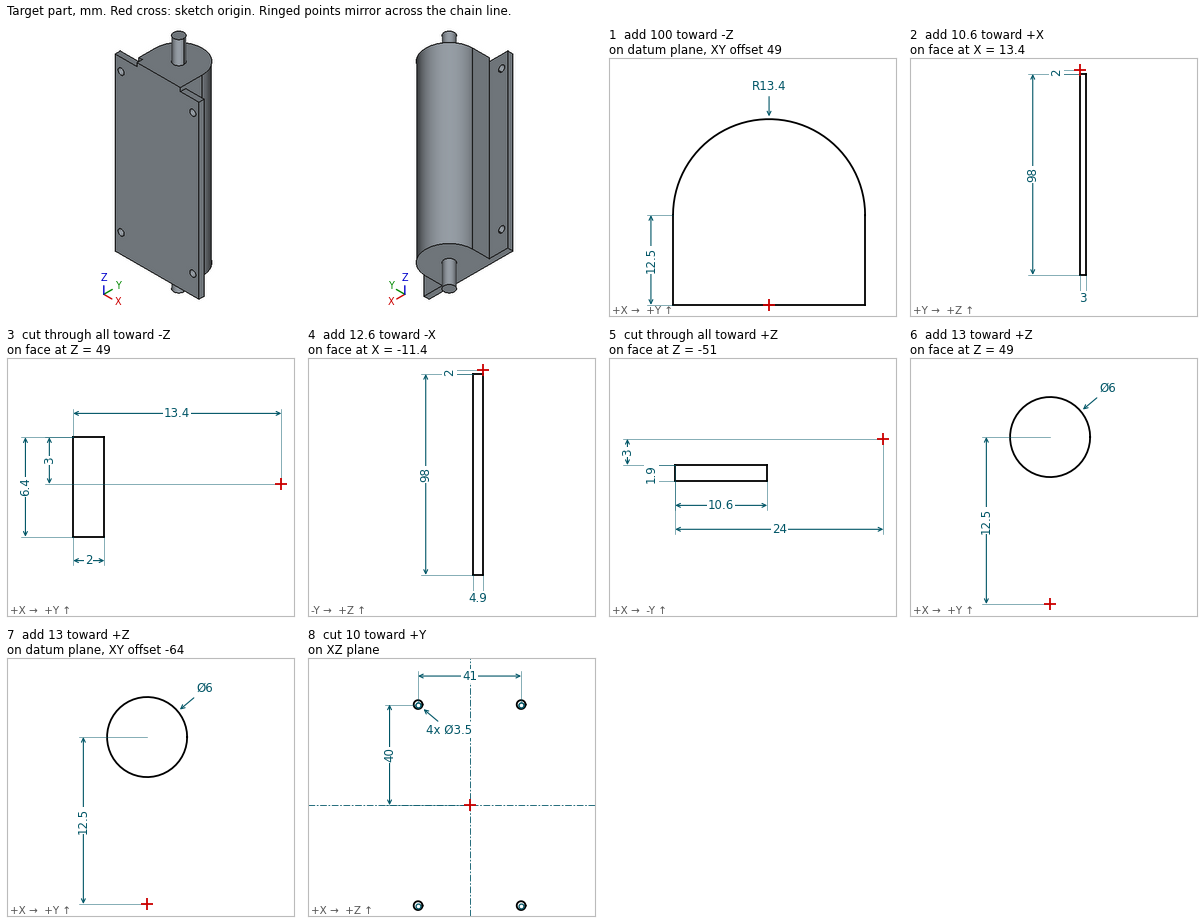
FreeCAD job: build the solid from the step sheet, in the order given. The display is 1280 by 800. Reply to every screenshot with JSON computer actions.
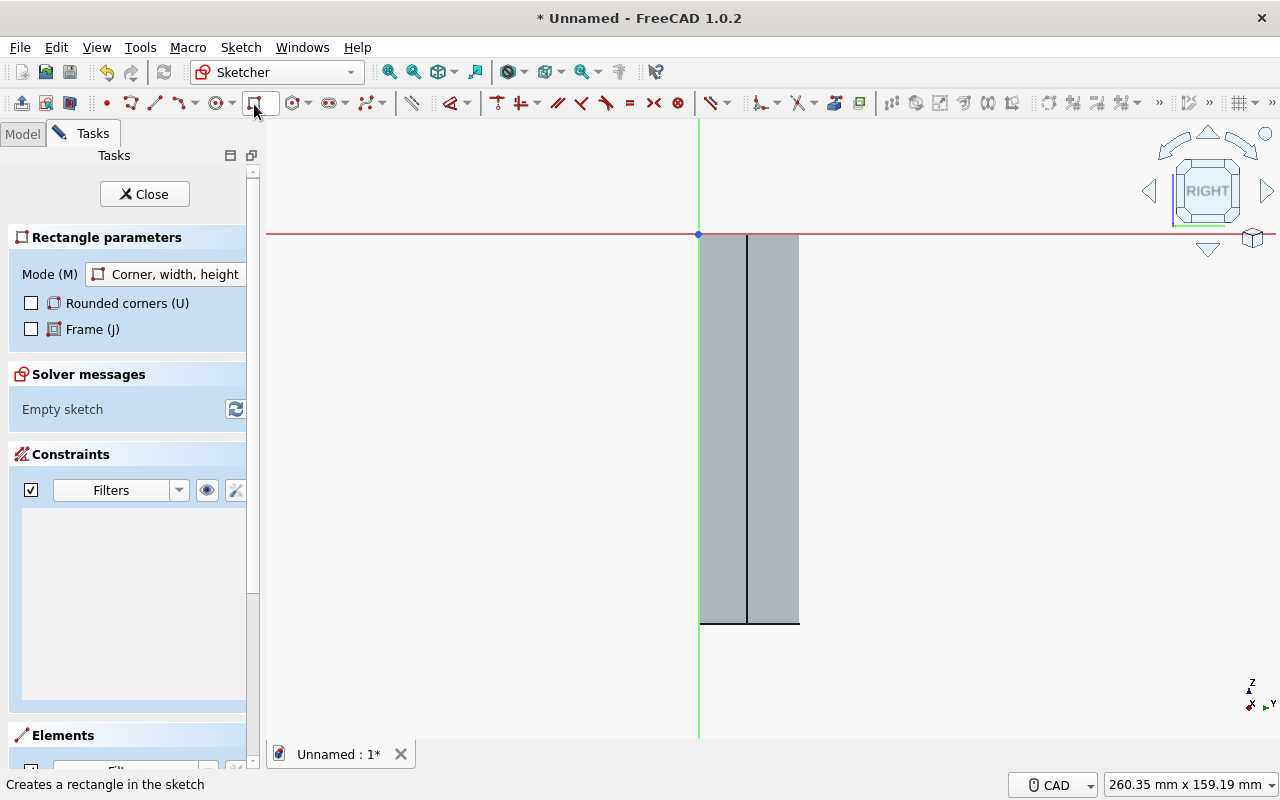
{"action": "scroll", "coordinate": [699, 242], "scroll_direction": "up", "scroll_amount": 4}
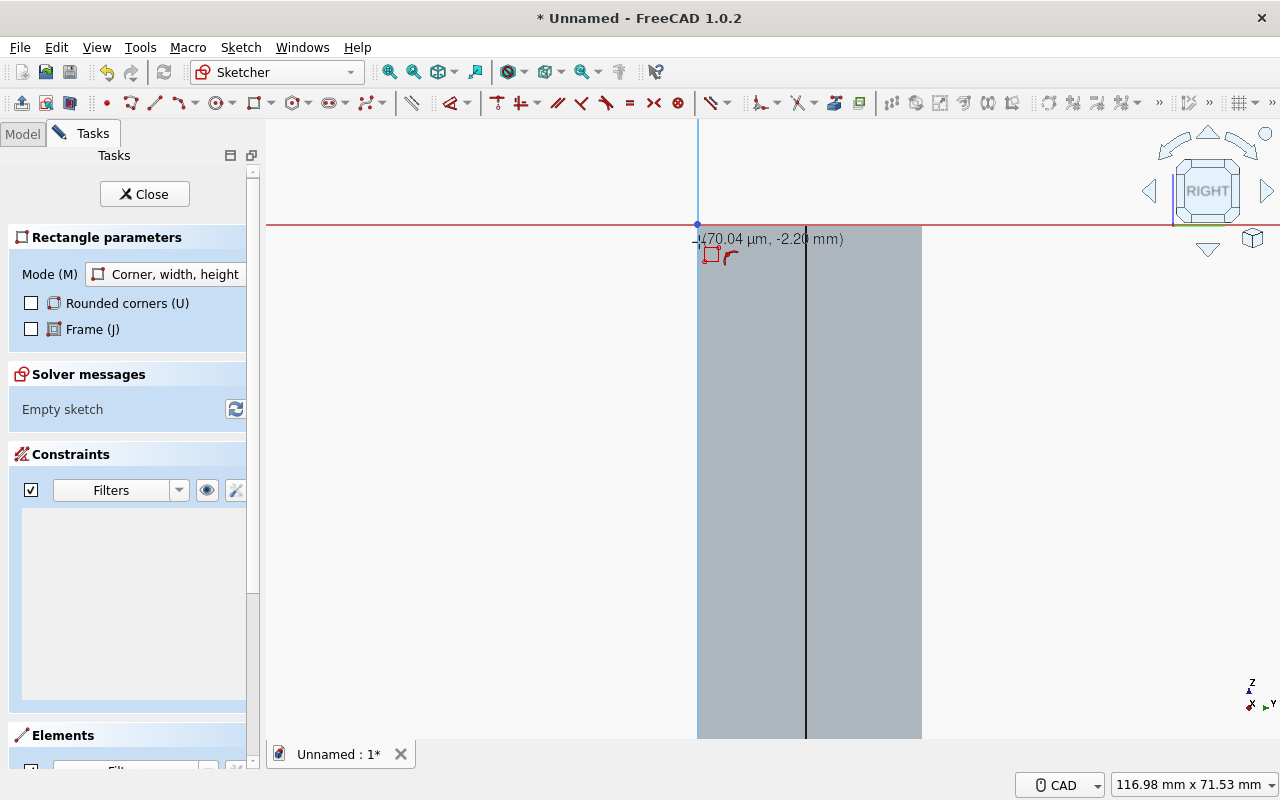
{"action": "left_click", "coordinate": [698, 242]}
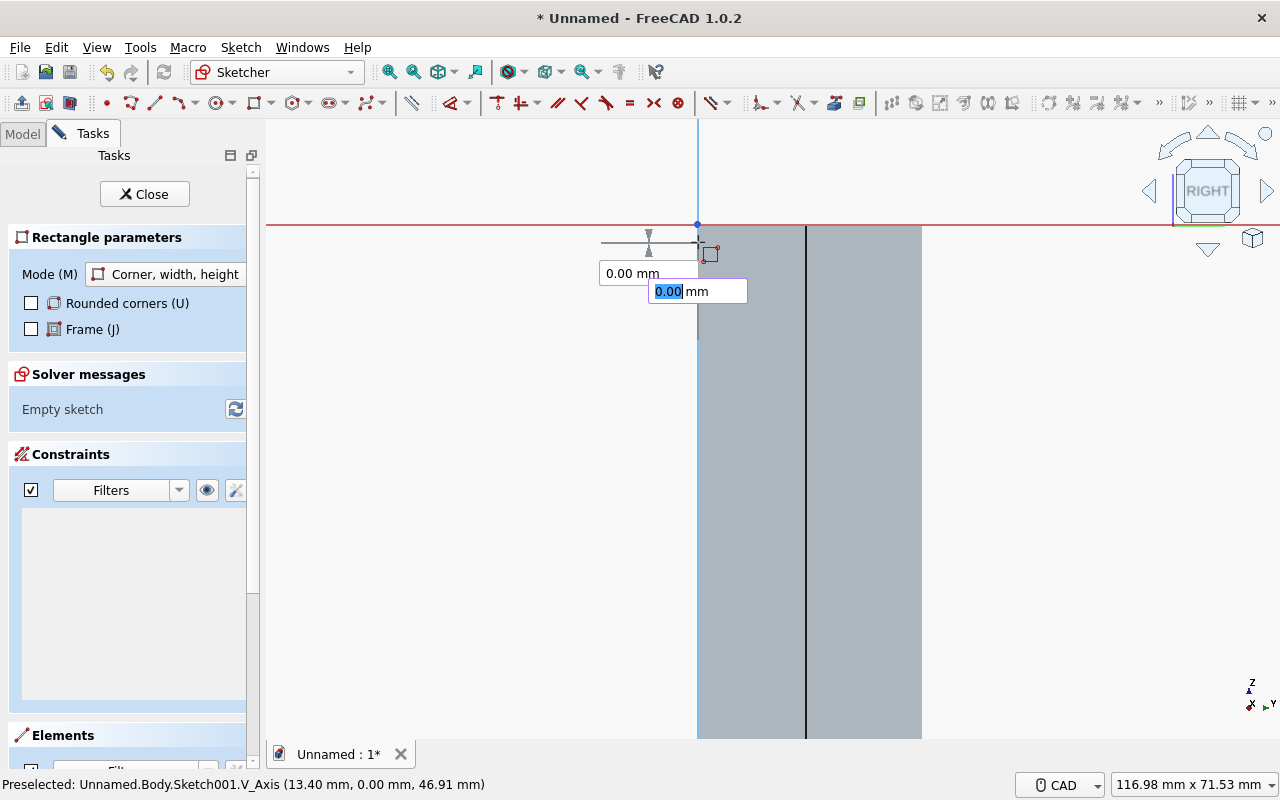
{"action": "scroll", "coordinate": [699, 242], "scroll_direction": "down", "scroll_amount": 4}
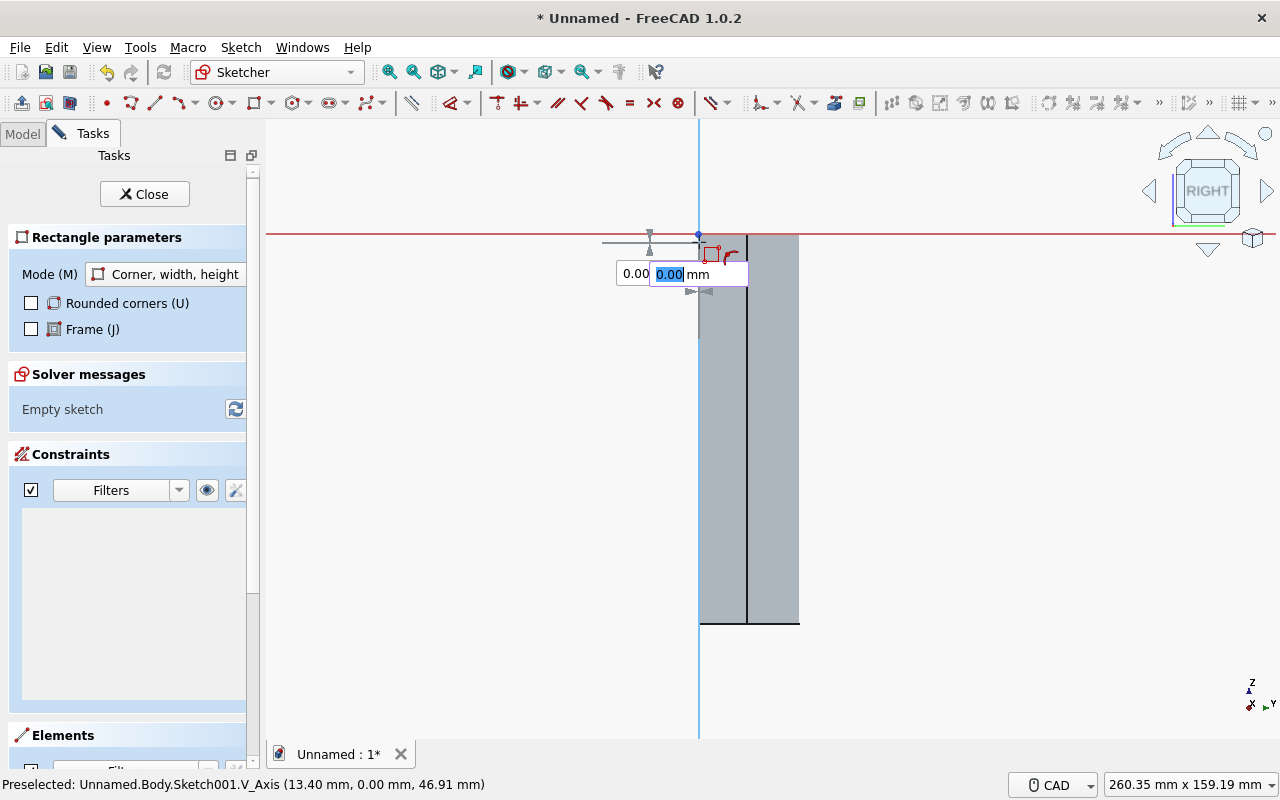
{"action": "scroll", "coordinate": [710, 624], "scroll_direction": "up", "scroll_amount": 2}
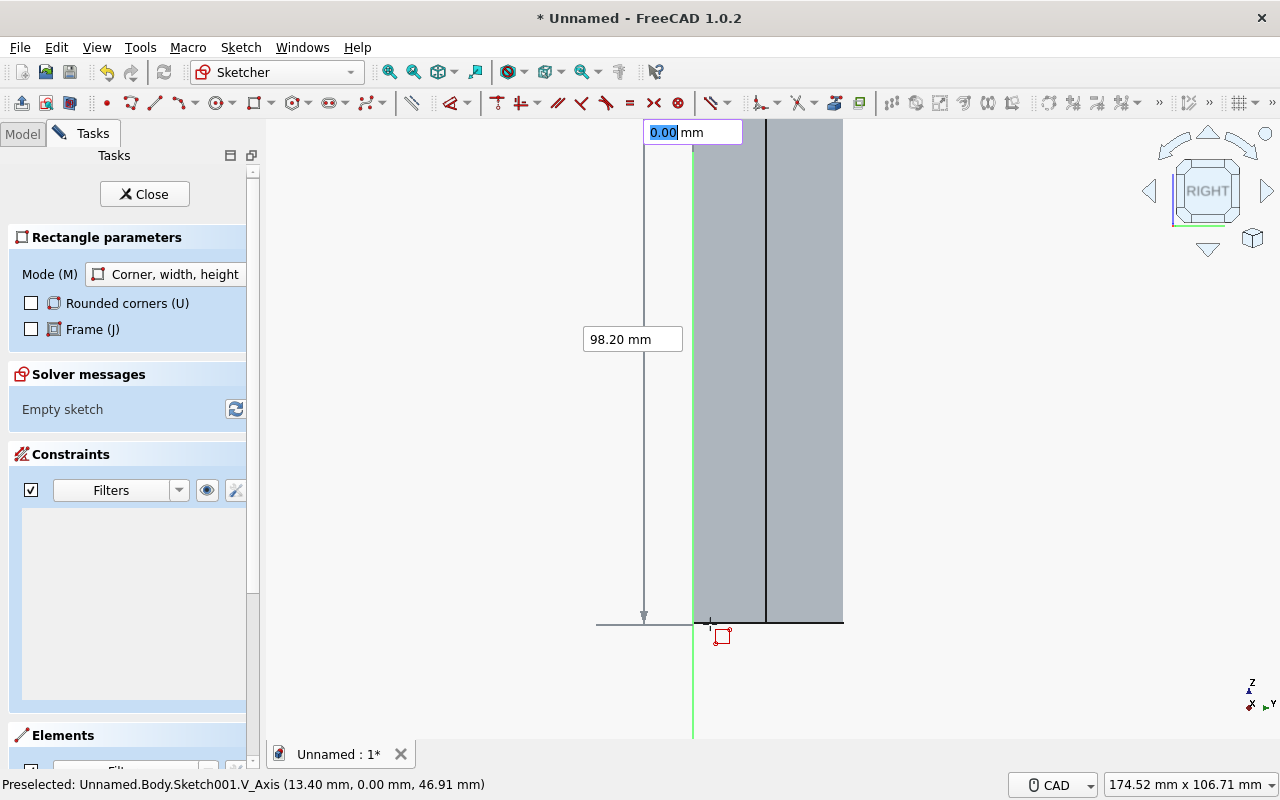
{"action": "left_click", "coordinate": [710, 623]}
{"action": "key", "text": "Escape"}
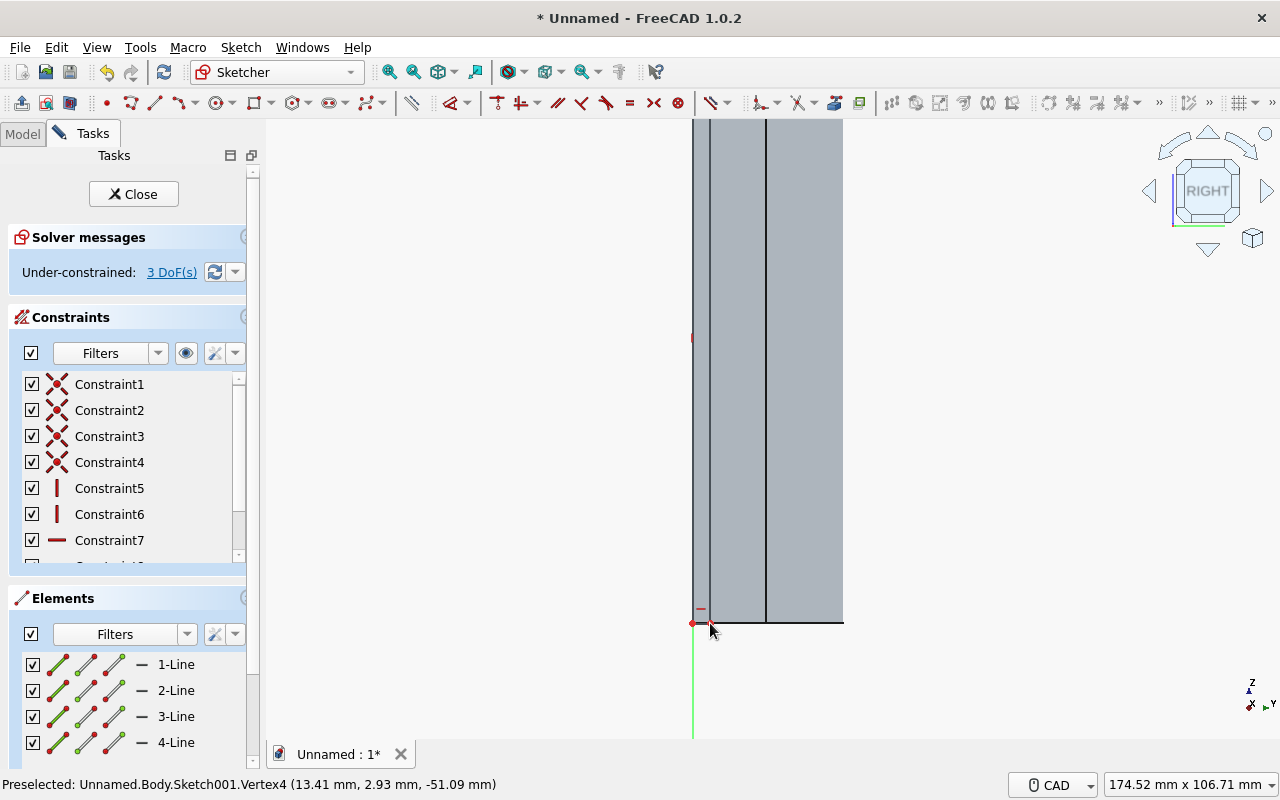
{"action": "left_click", "coordinate": [450, 104]}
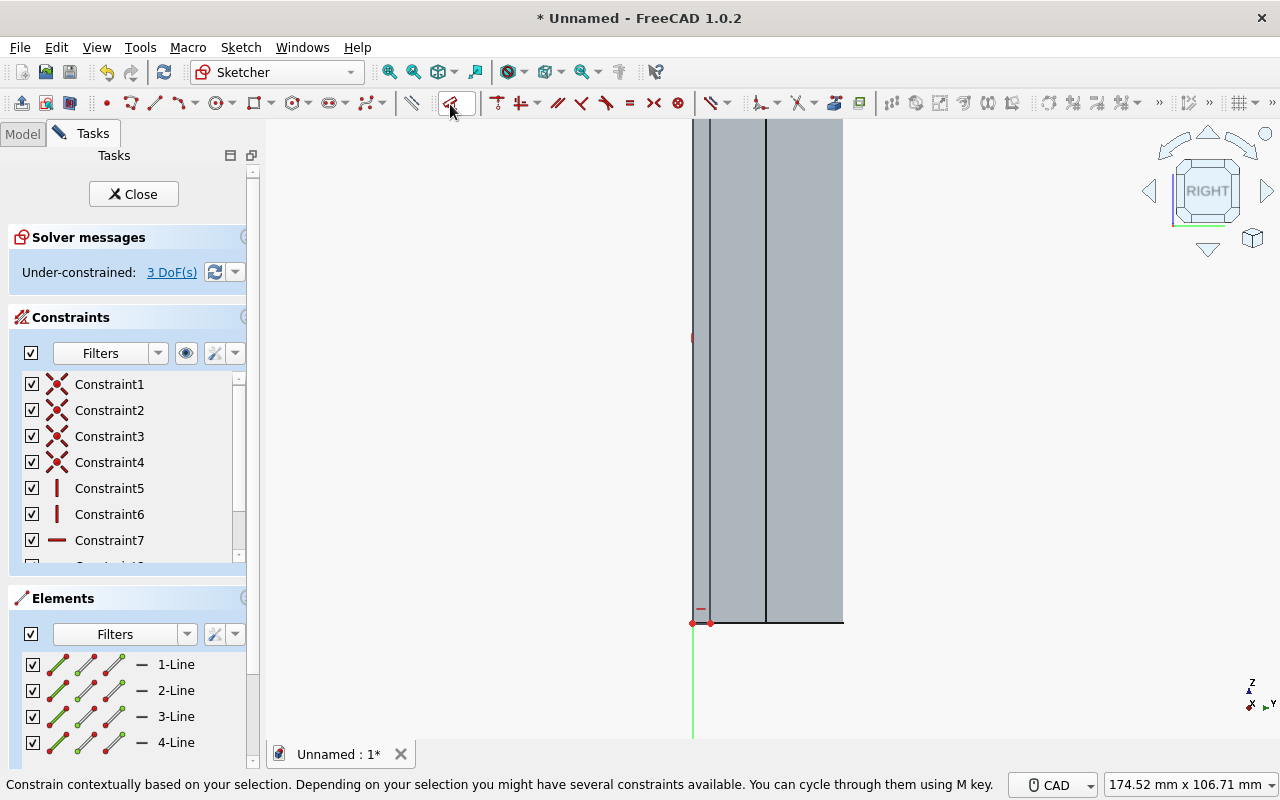
{"action": "scroll", "coordinate": [701, 624], "scroll_direction": "up", "scroll_amount": 5}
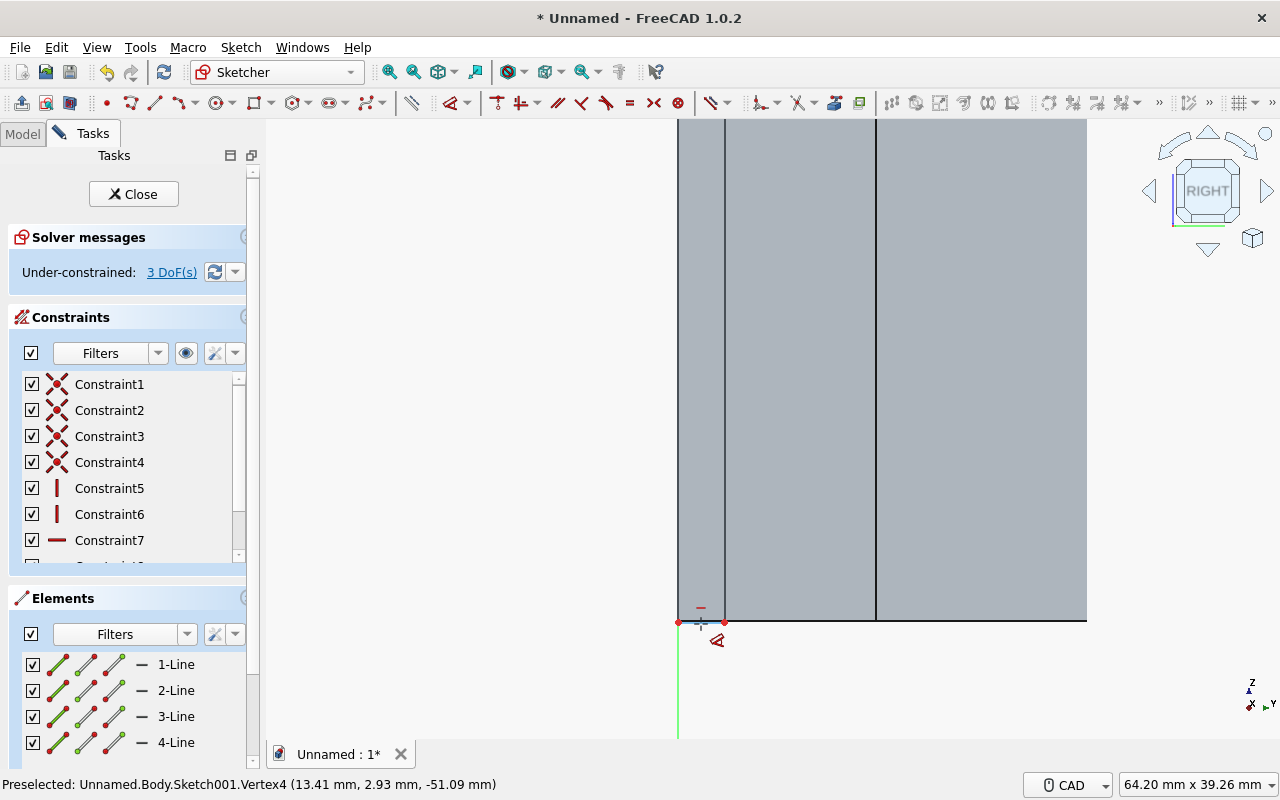
{"action": "left_click", "coordinate": [702, 623]}
{"action": "left_click", "coordinate": [702, 657]}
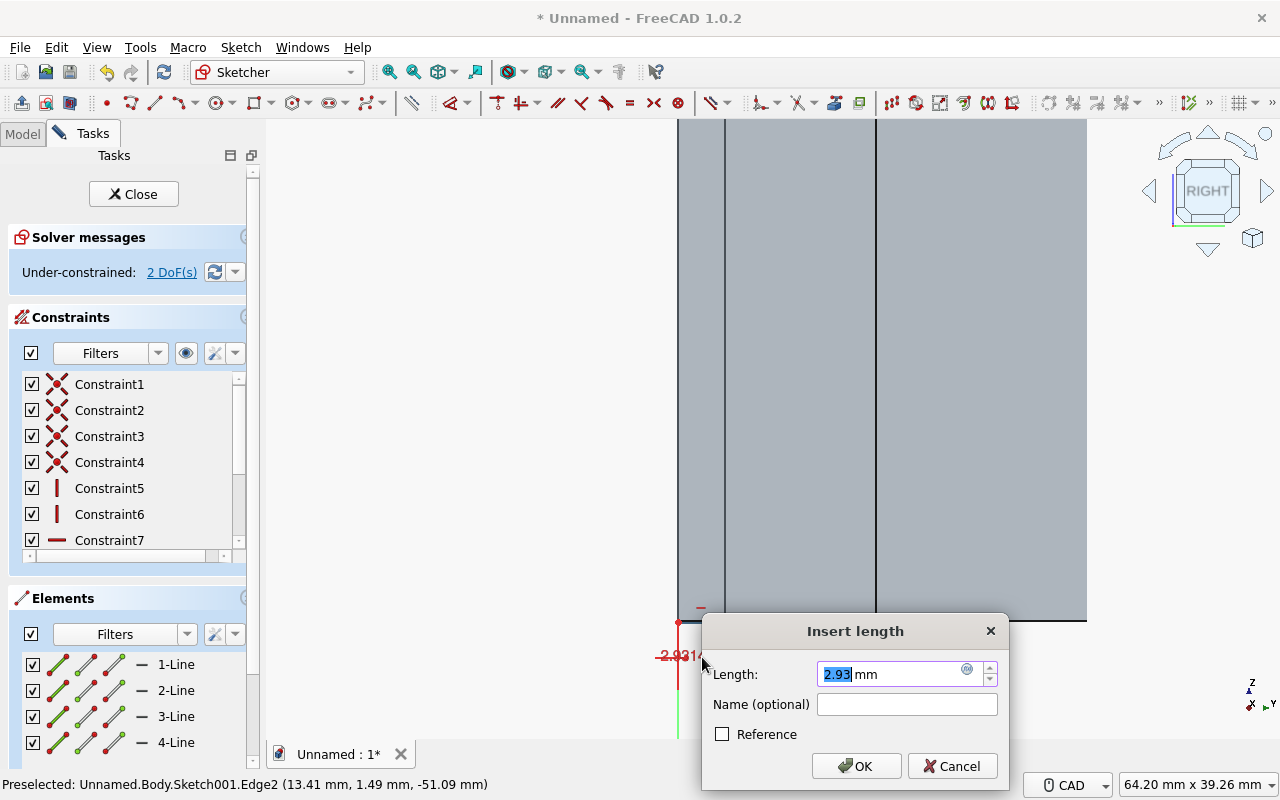
{"action": "type", "text": "3"}
{"action": "key", "text": "Return"}